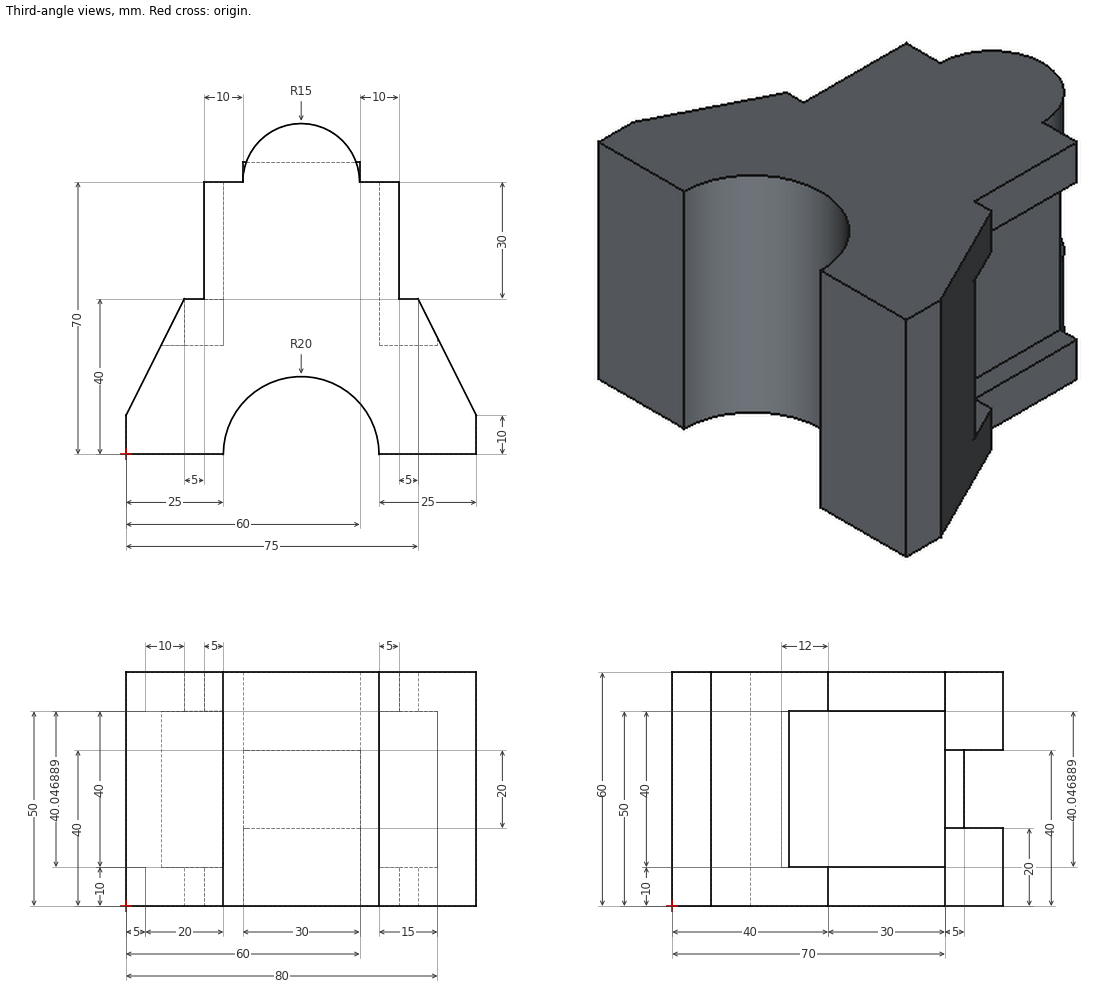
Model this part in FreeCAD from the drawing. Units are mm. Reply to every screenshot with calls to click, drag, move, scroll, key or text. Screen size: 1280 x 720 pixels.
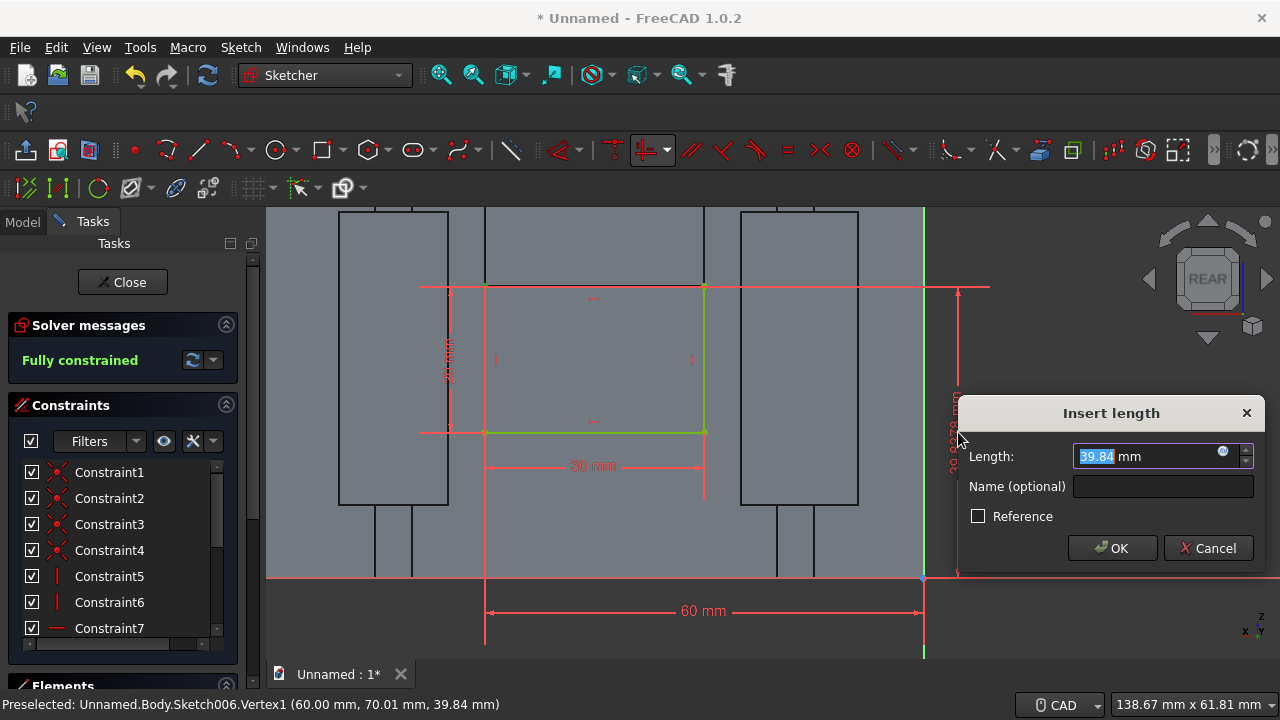
text(40)
key(Return)
key(Escape)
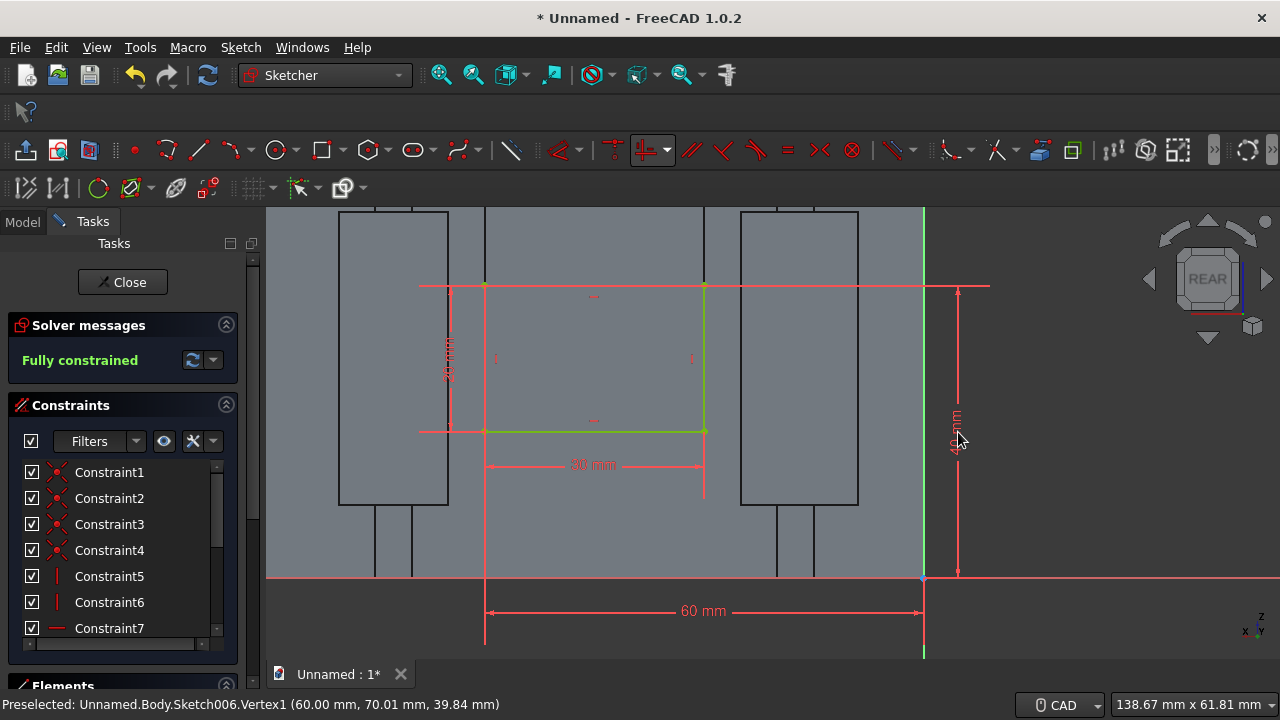
click(123, 282)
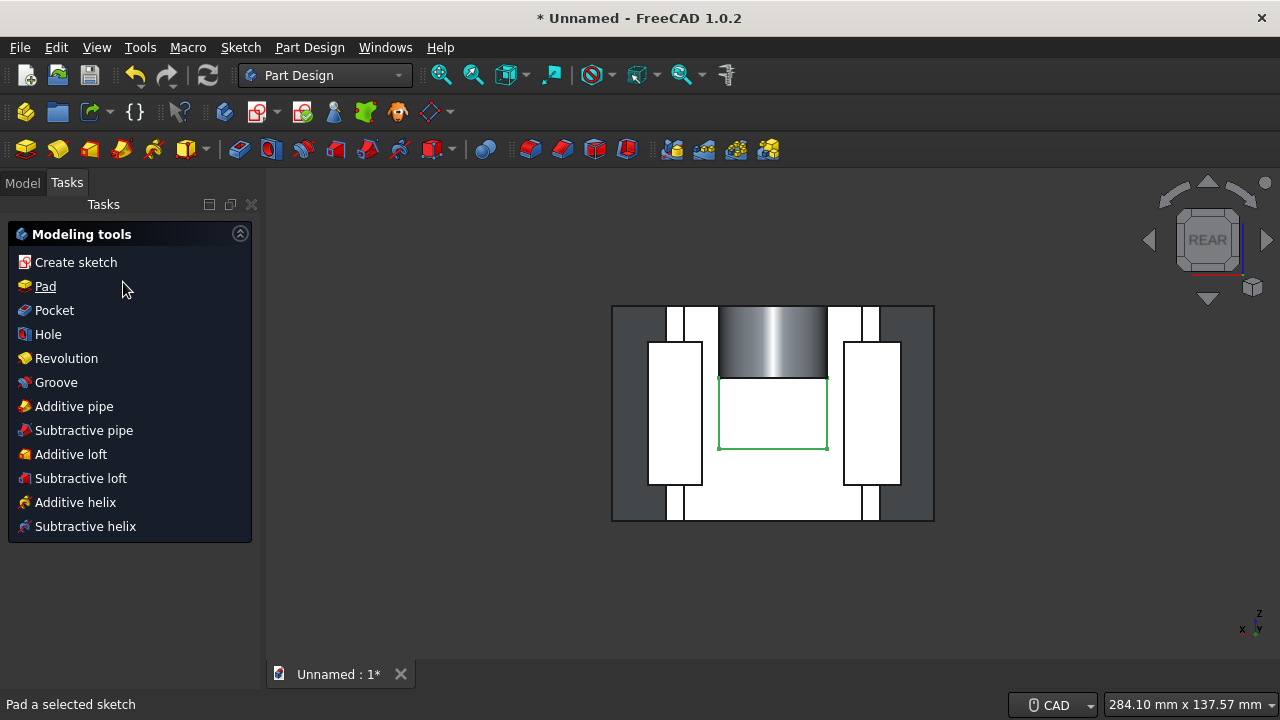
click(26, 150)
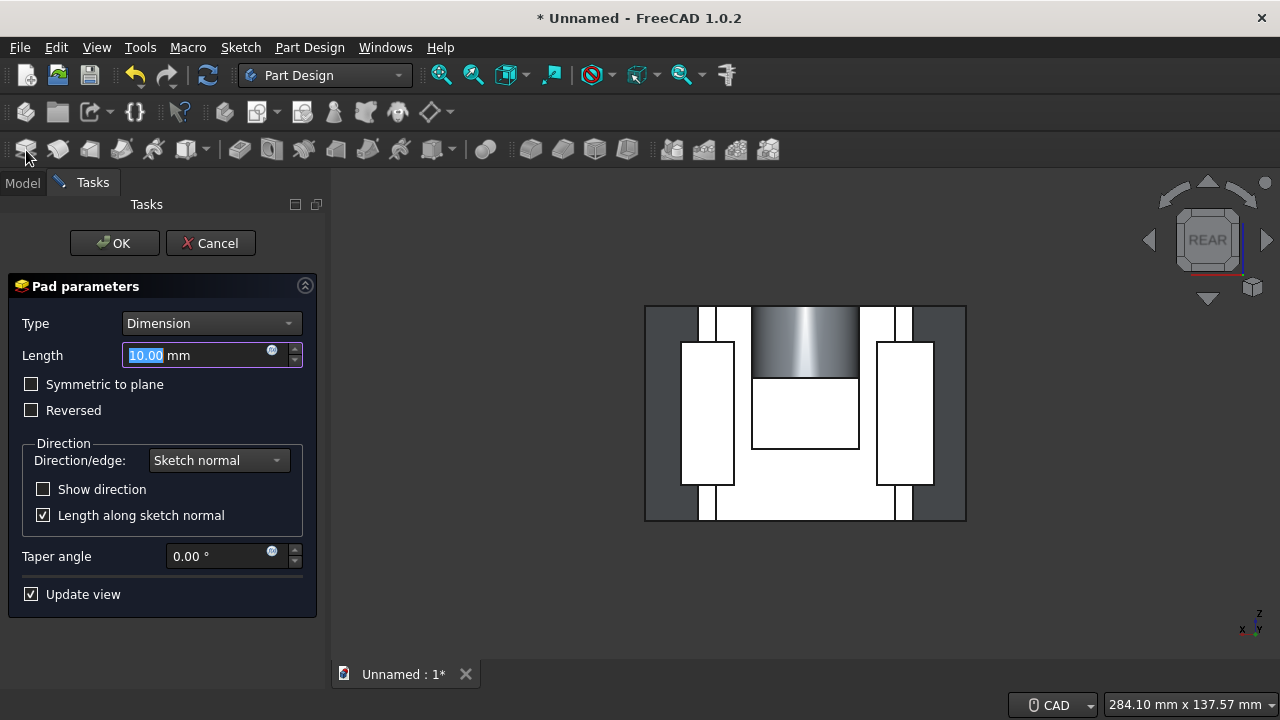
text(5)
key(Tab)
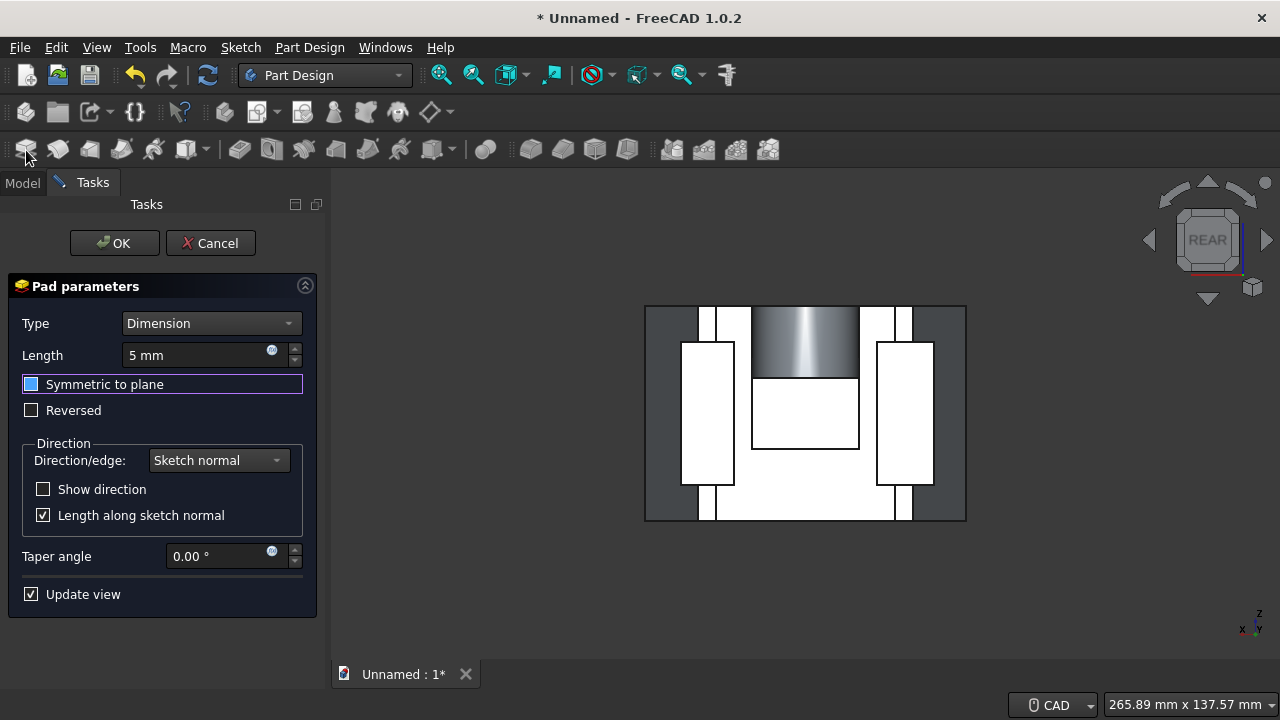
click(115, 243)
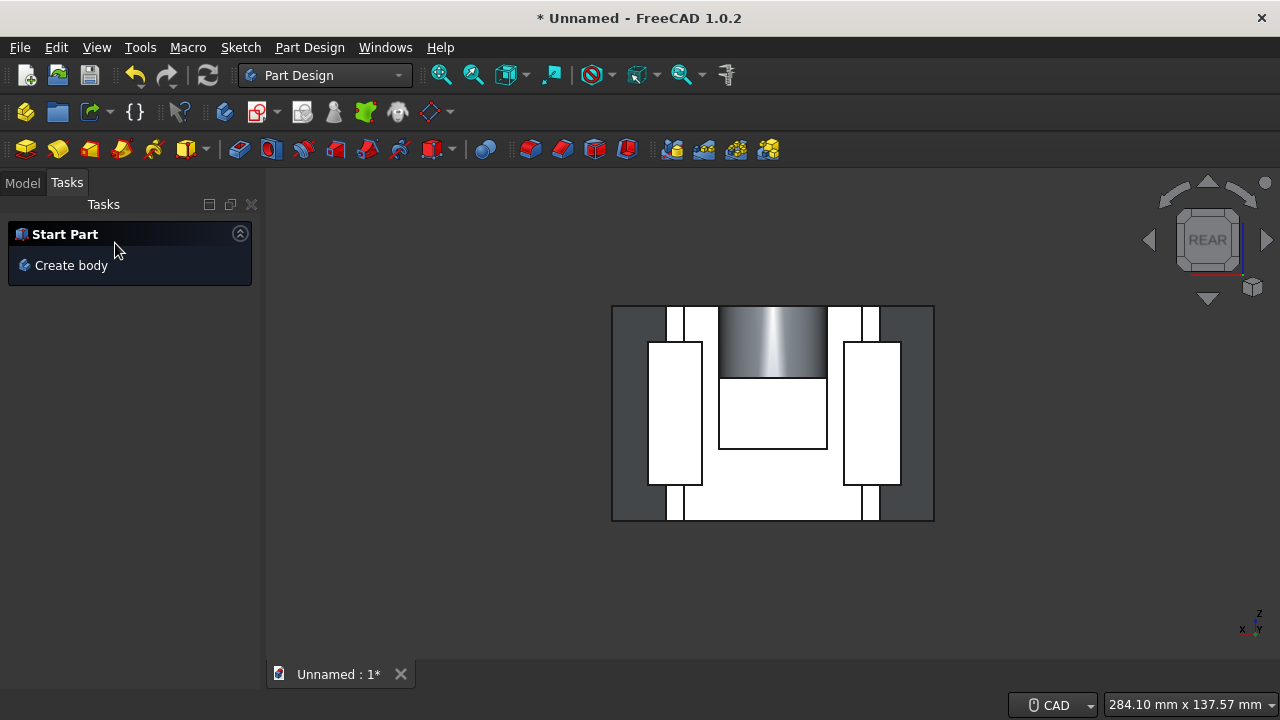
click(442, 76)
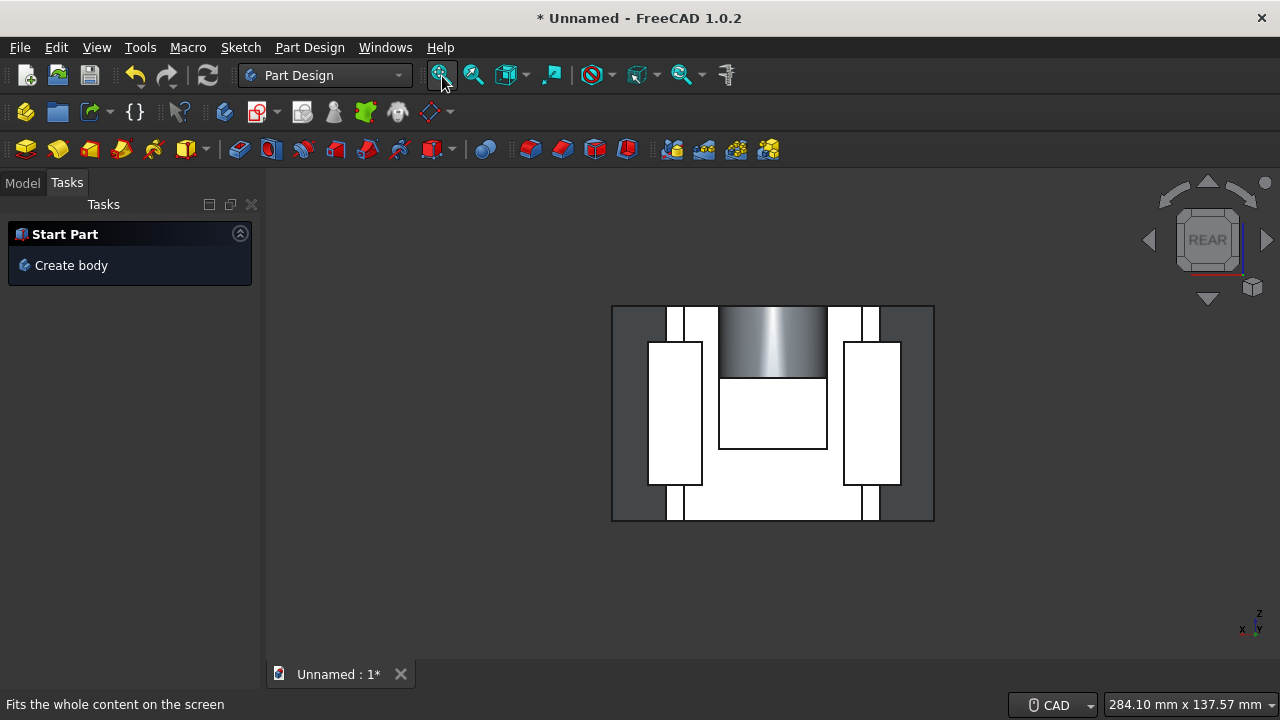
click(258, 112)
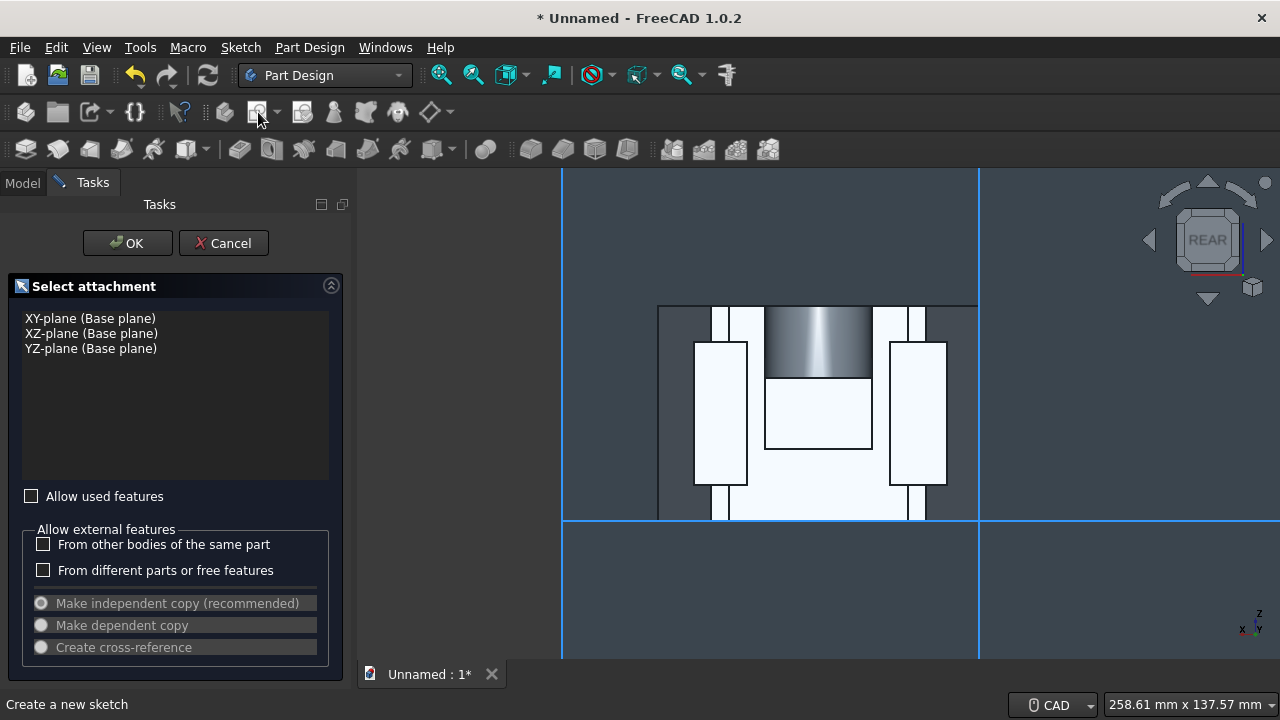
click(82, 318)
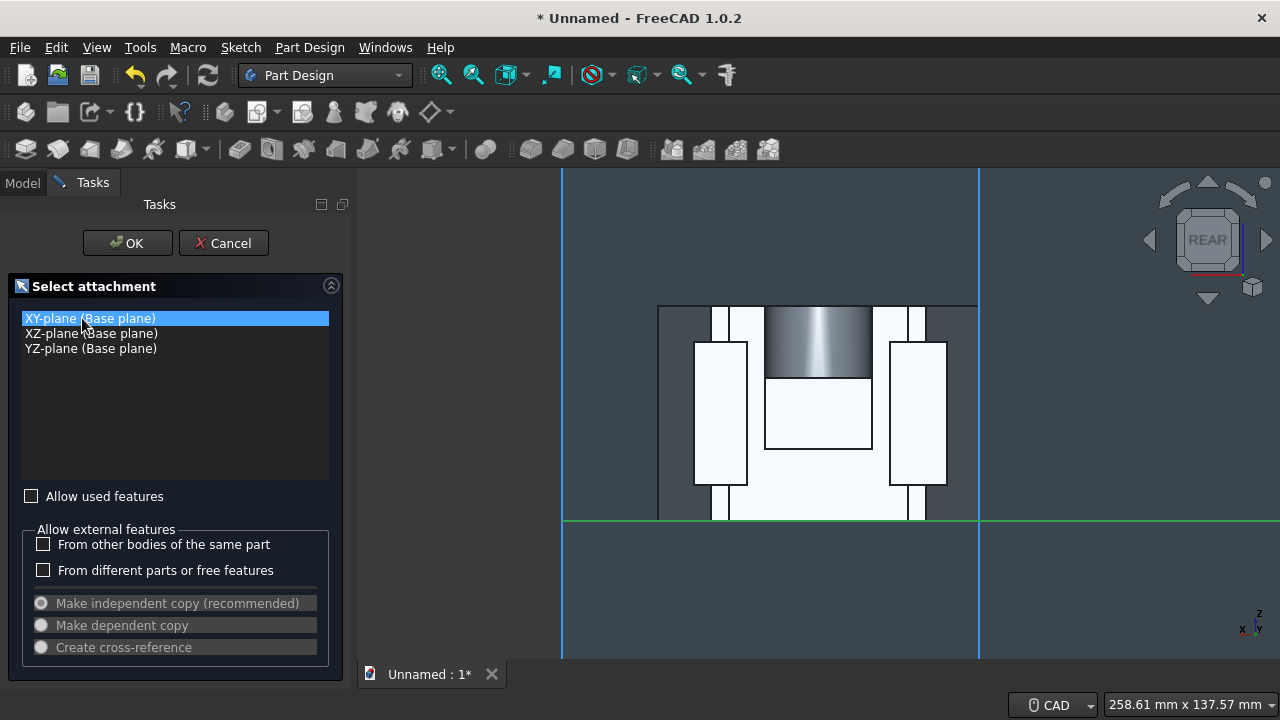
click(128, 243)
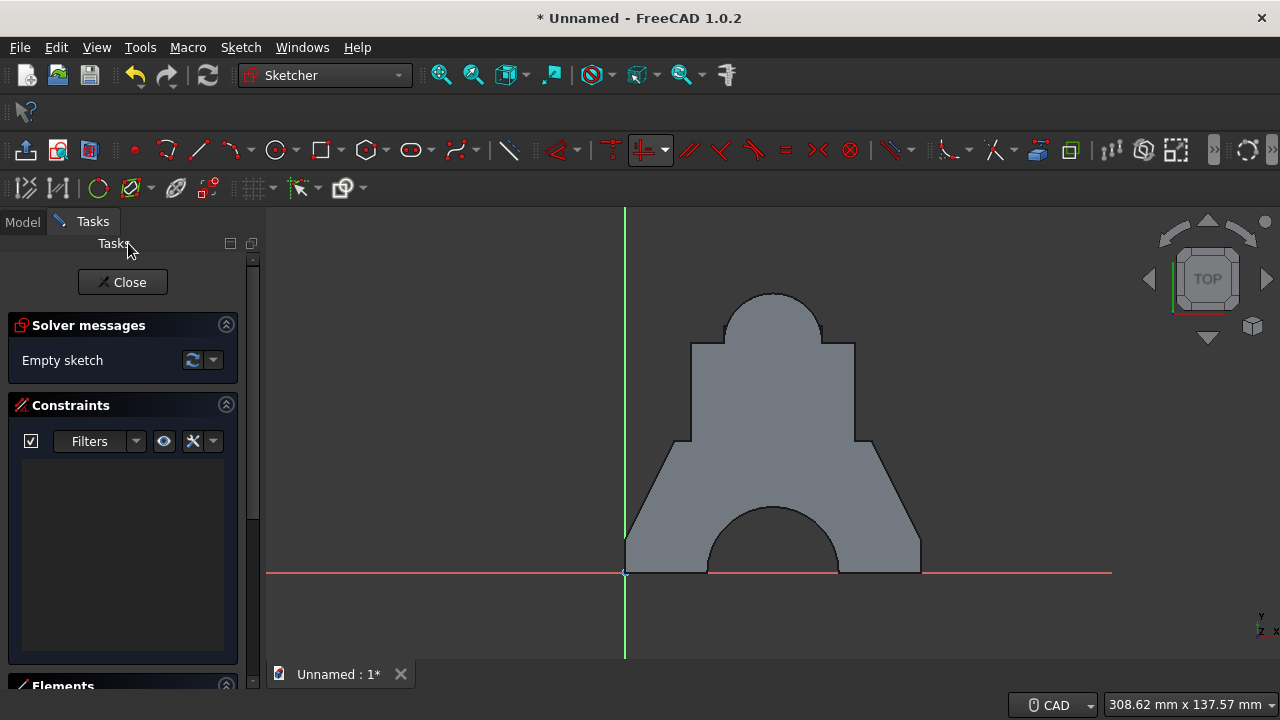
click(90, 150)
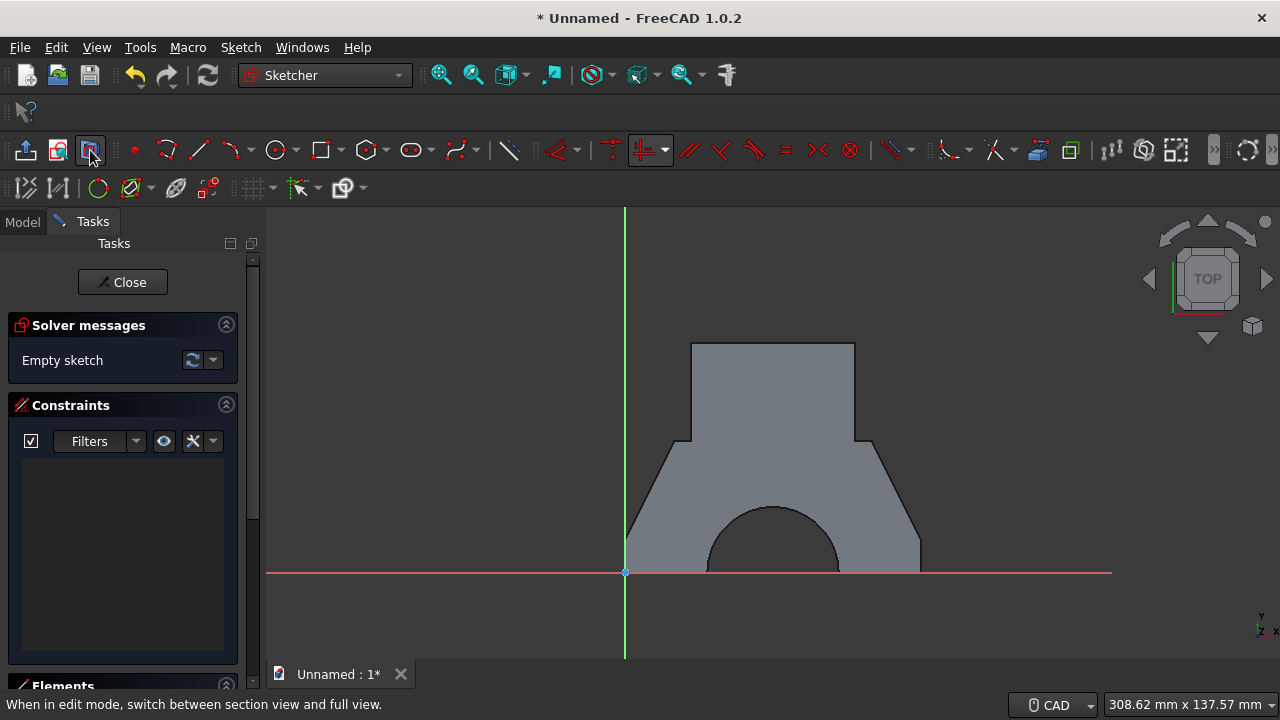
scroll(787, 295, up, 9)